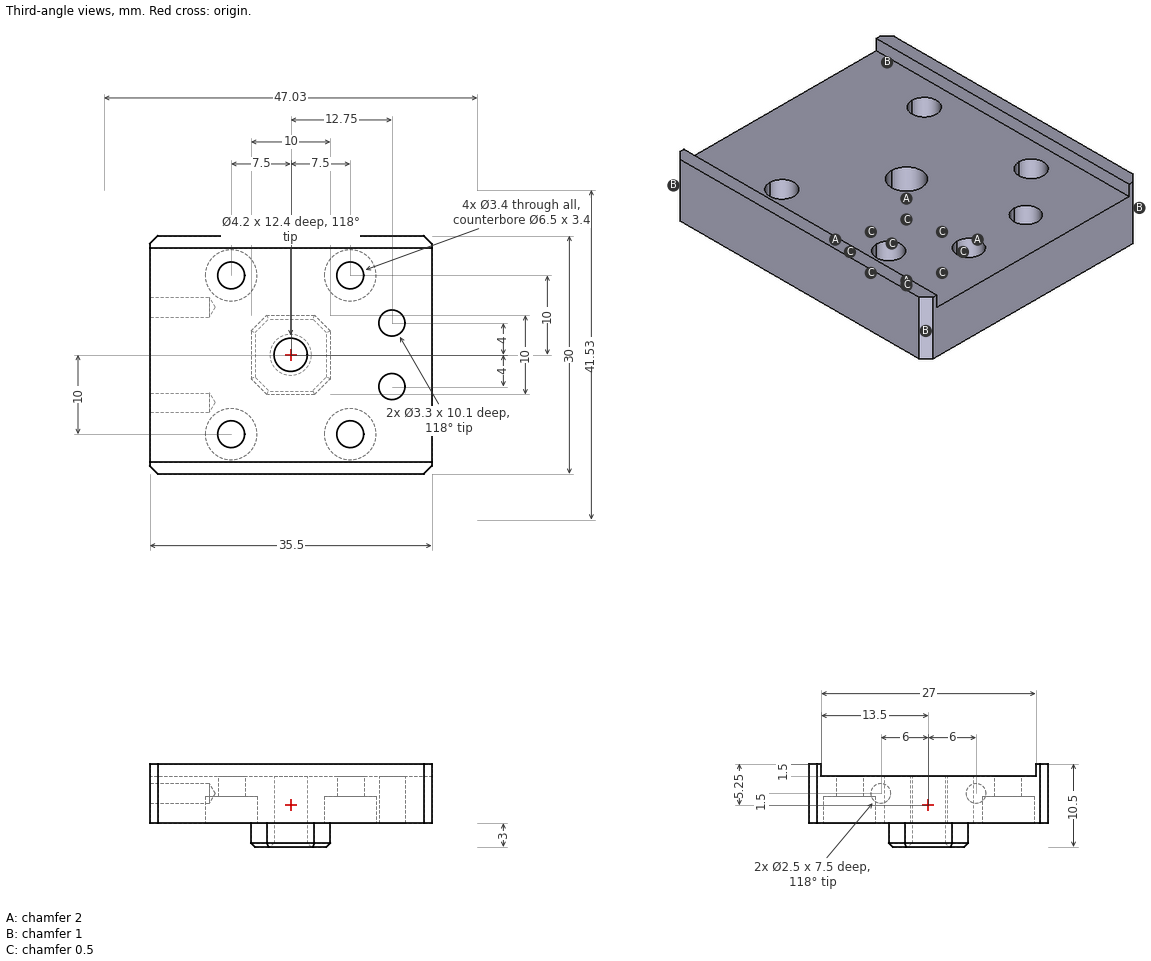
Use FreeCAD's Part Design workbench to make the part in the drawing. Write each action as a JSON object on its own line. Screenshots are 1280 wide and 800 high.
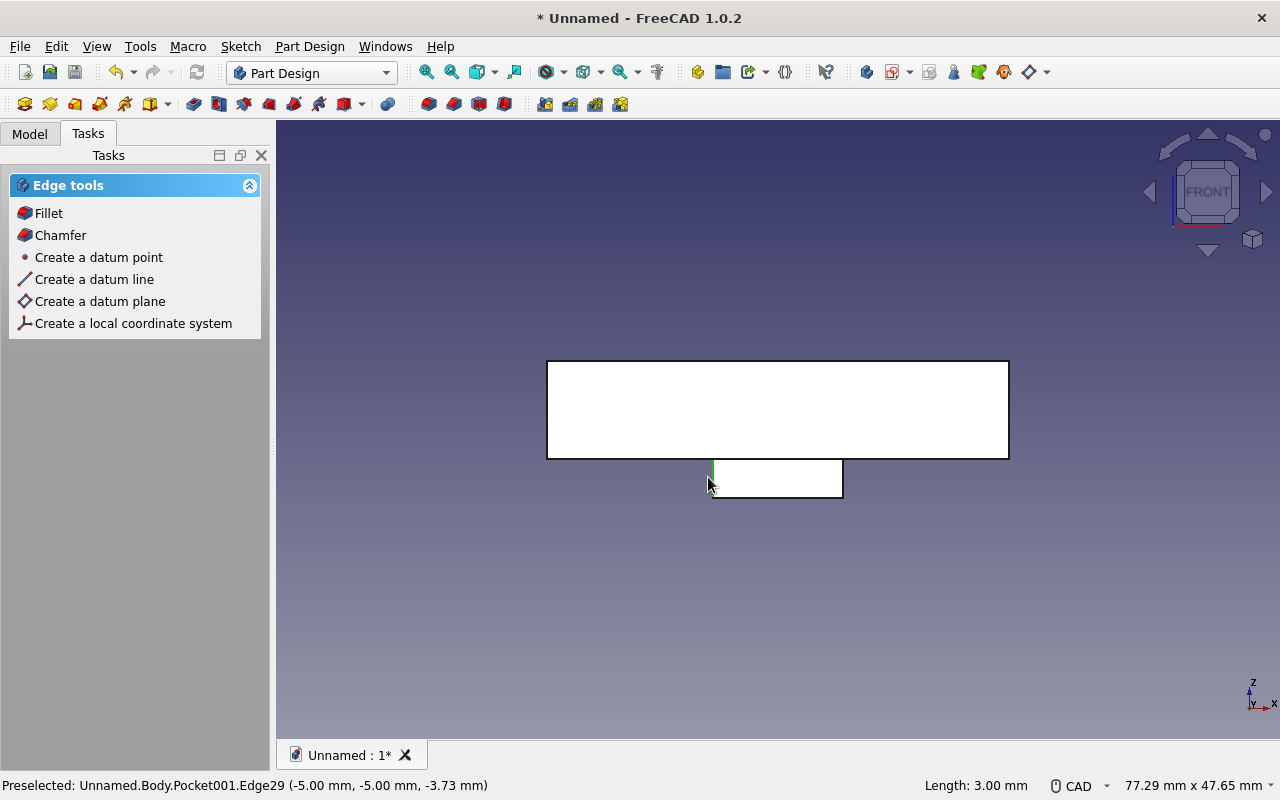
{"action": "left_click", "coordinate": [843, 477], "text": "ctrl"}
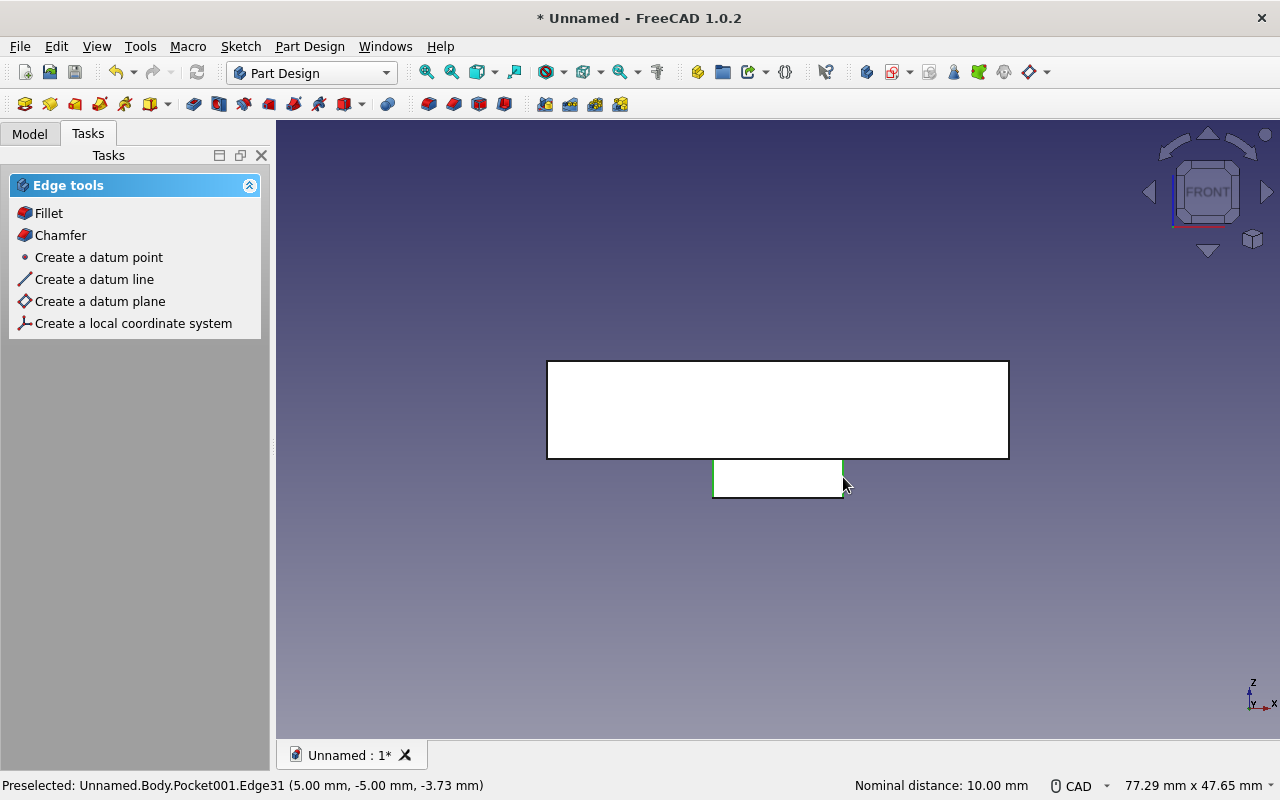
{"action": "key", "text": "3"}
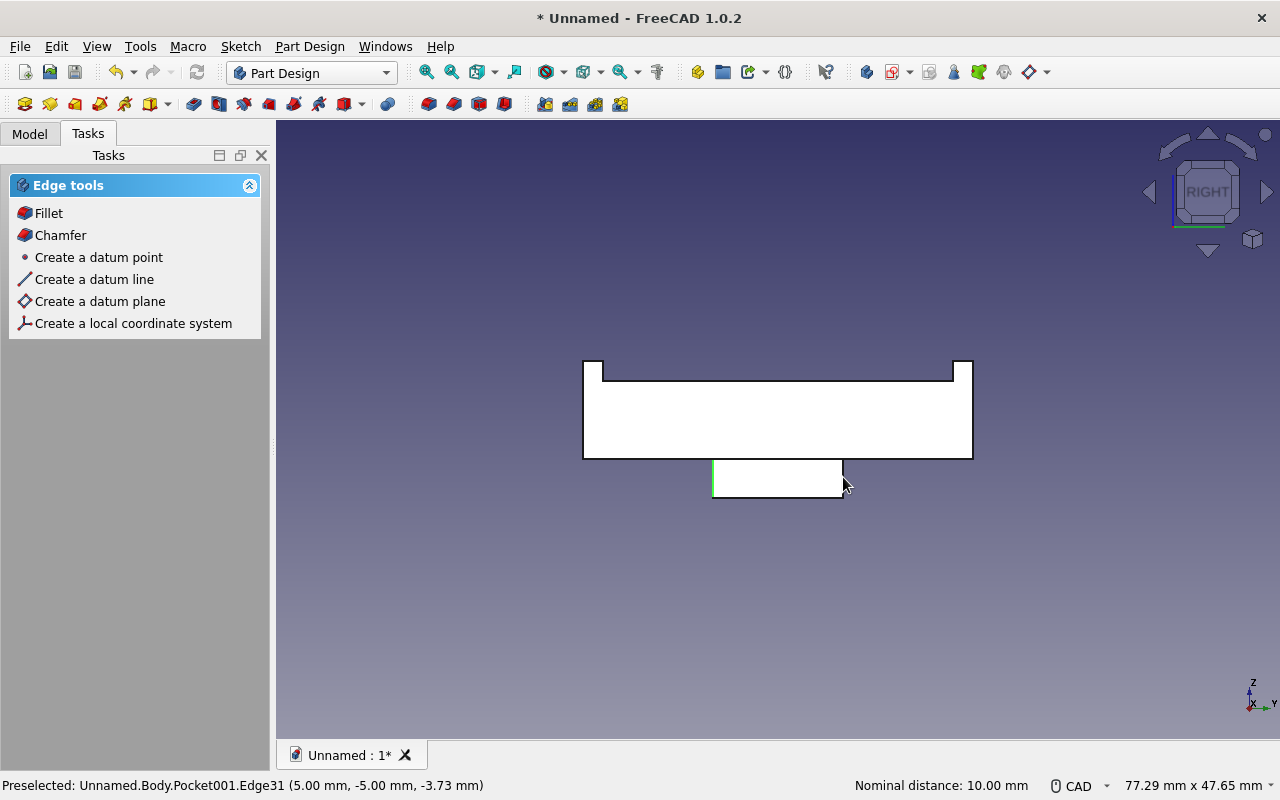
{"action": "key", "text": "v f"}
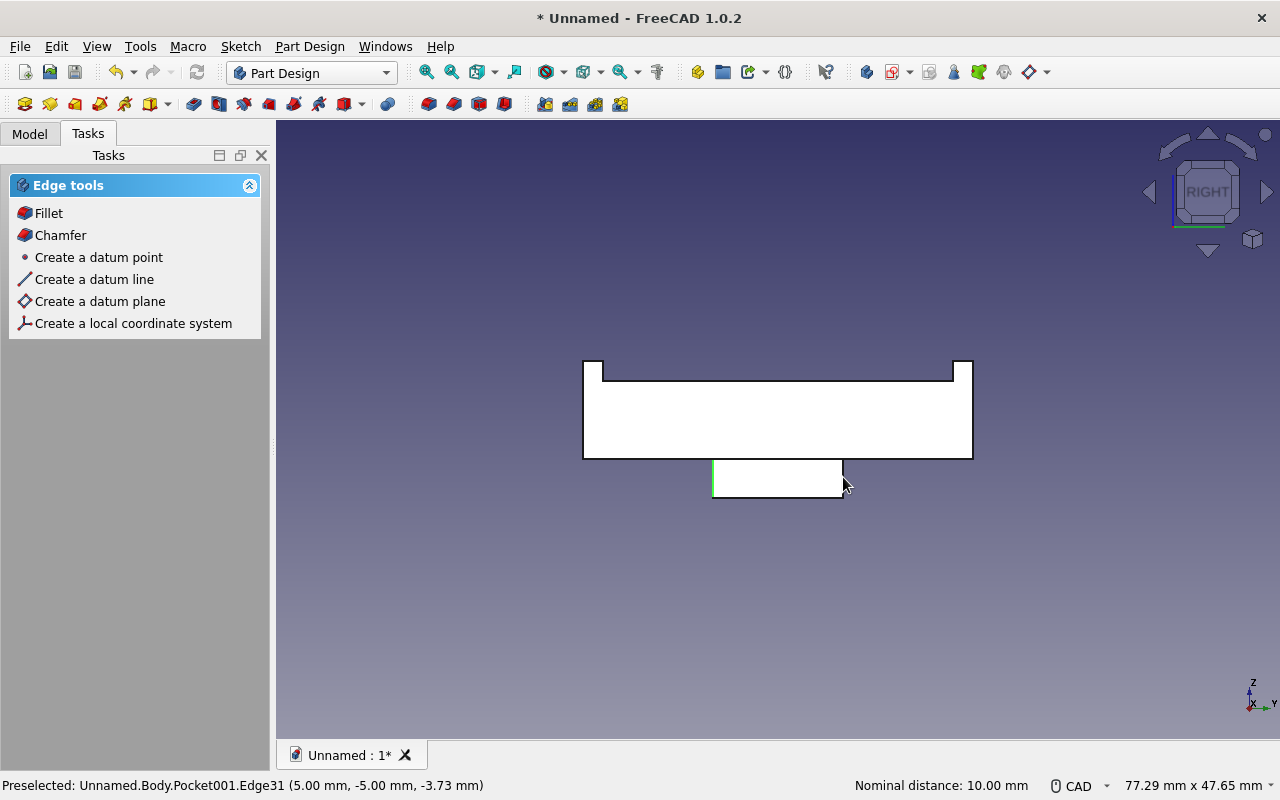
{"action": "left_click", "coordinate": [843, 477], "text": "ctrl"}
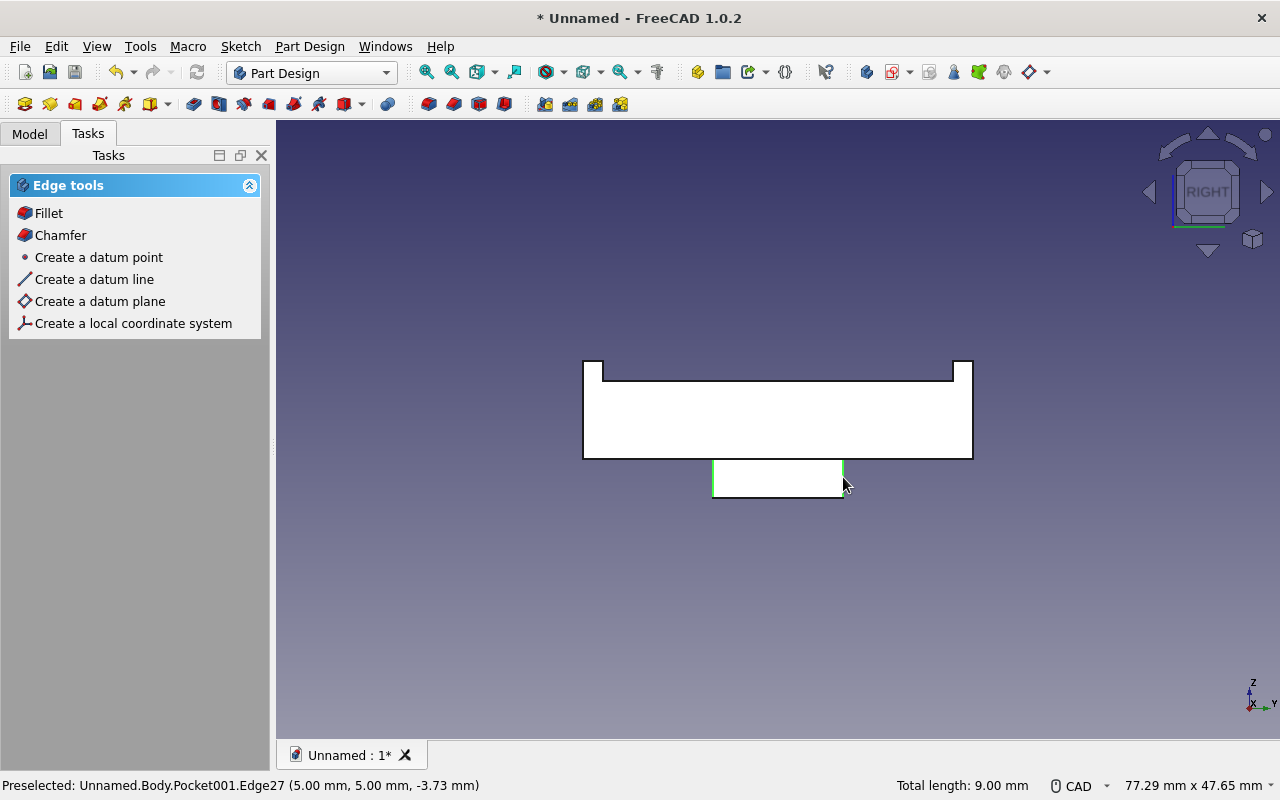
{"action": "key", "text": "5"}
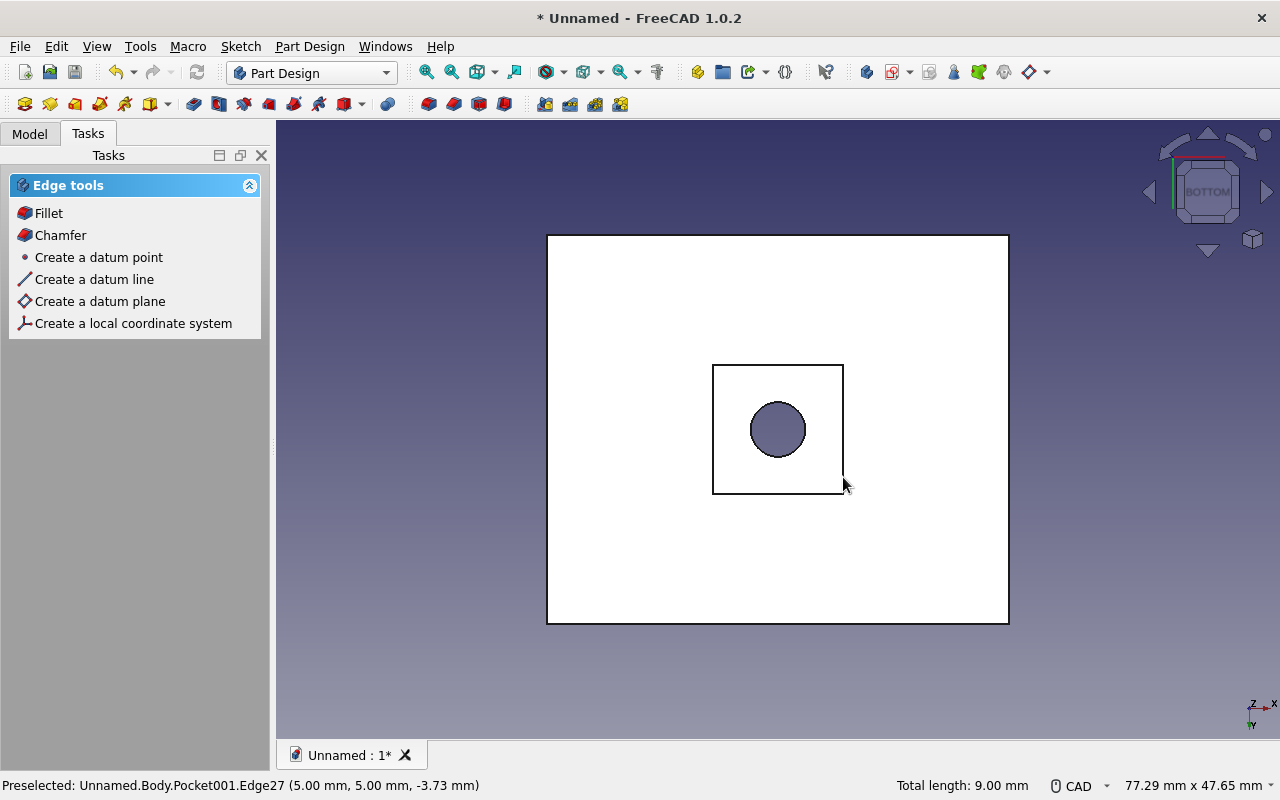
{"action": "key", "text": "4"}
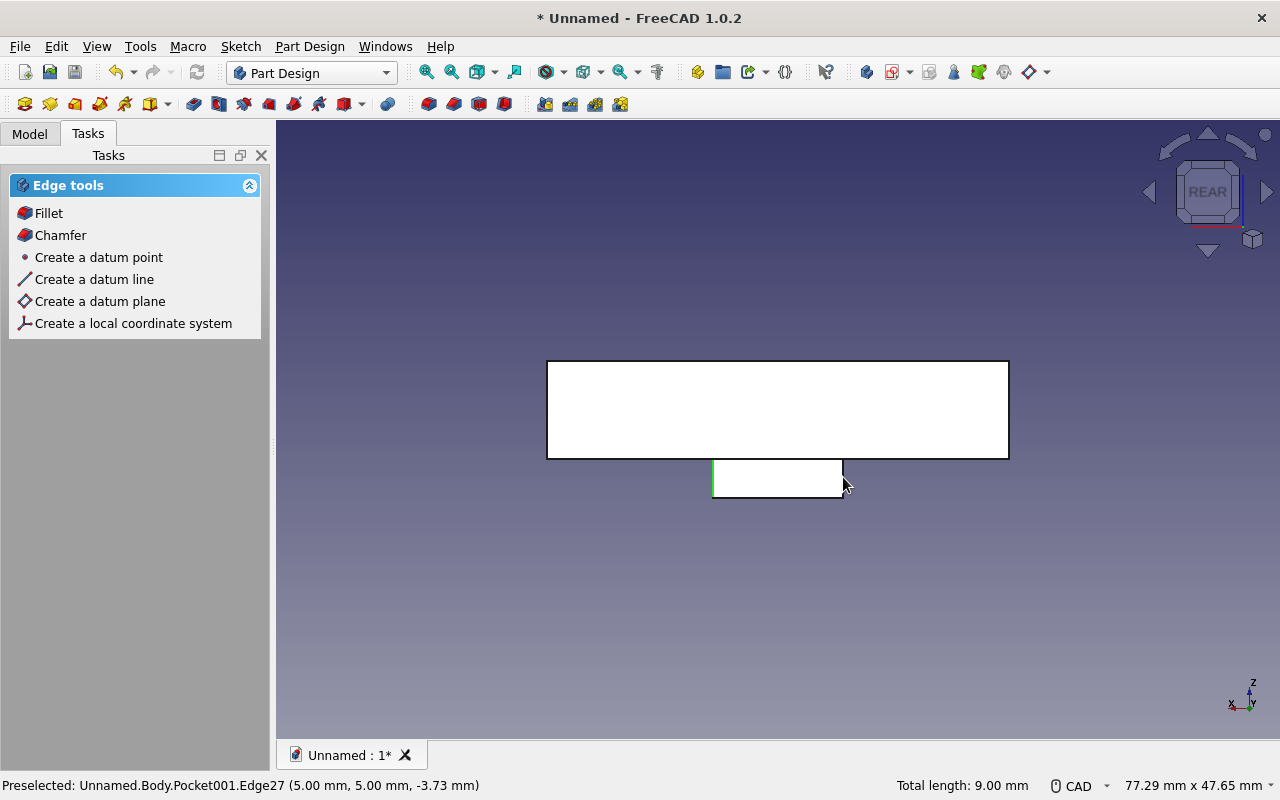
{"action": "left_click", "coordinate": [843, 477], "text": "ctrl"}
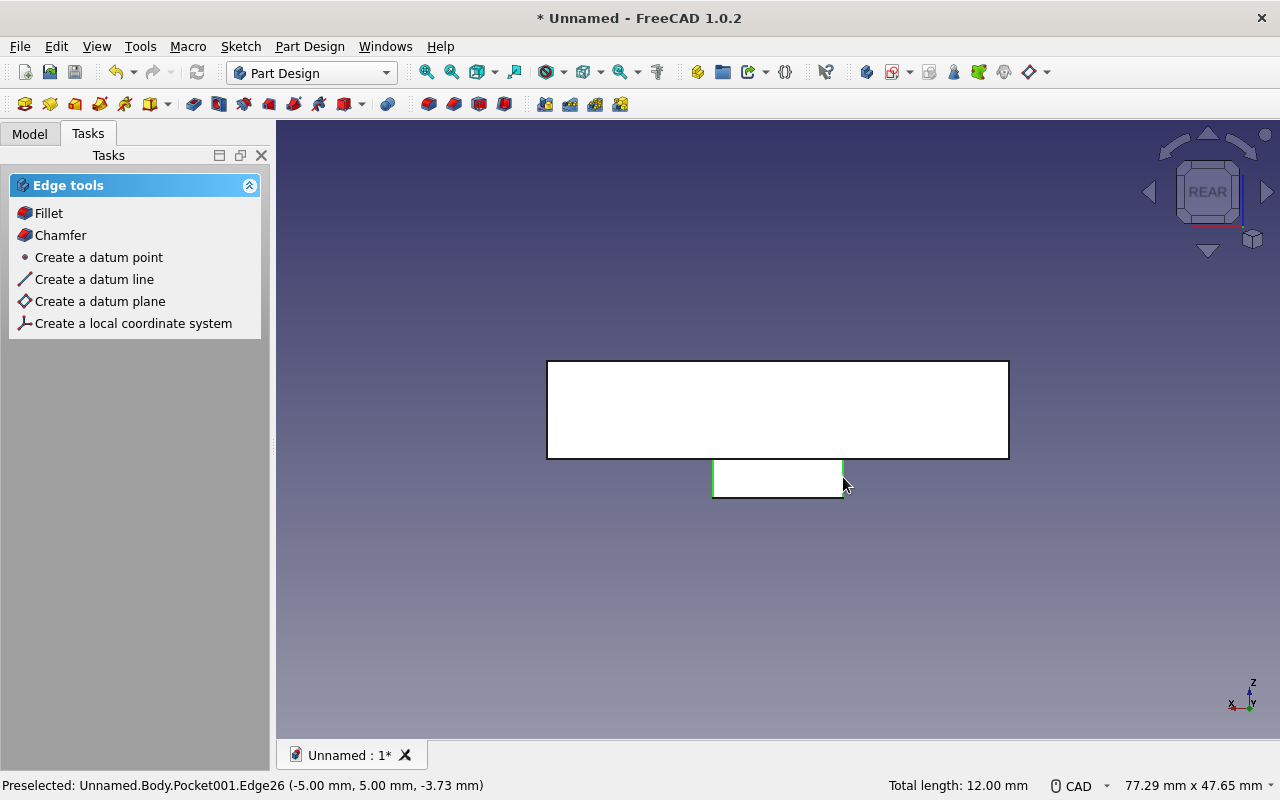
{"action": "left_click", "coordinate": [454, 104]}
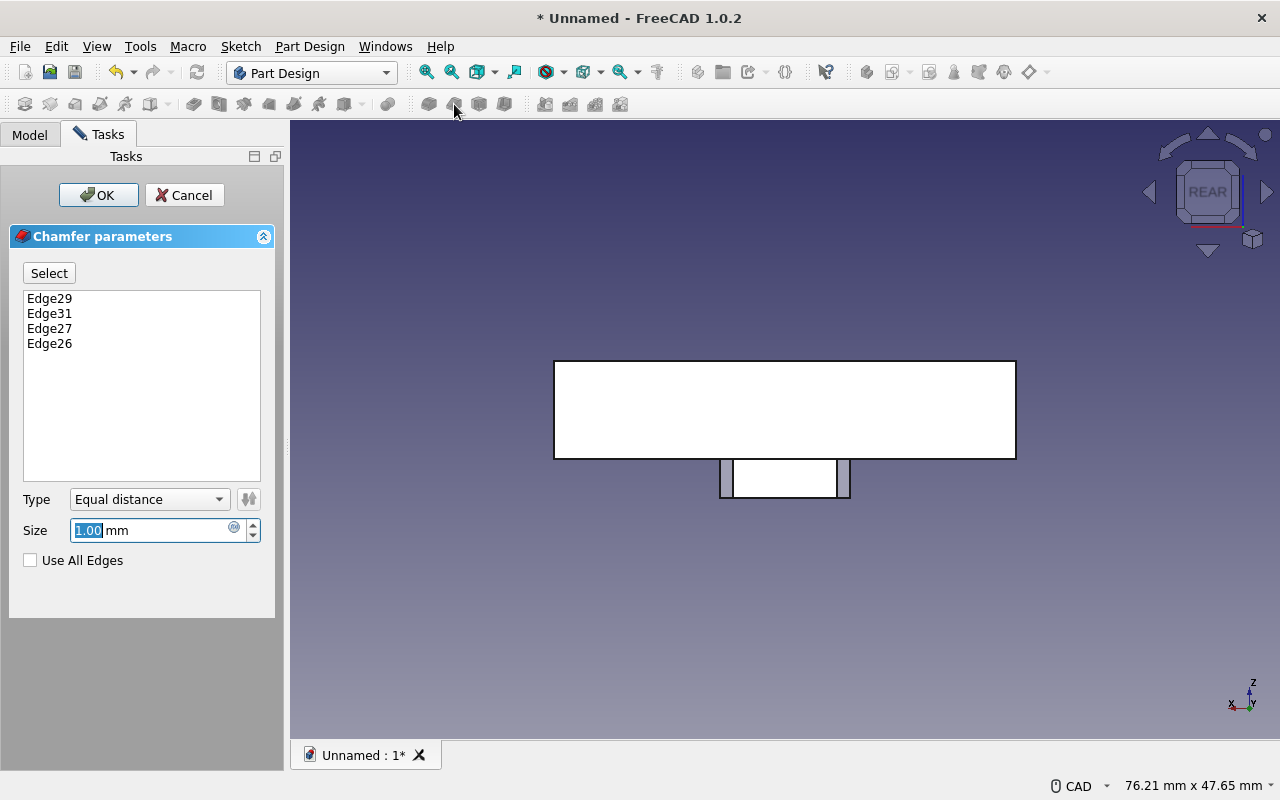
{"action": "type", "text": "2"}
{"action": "key", "text": "Tab"}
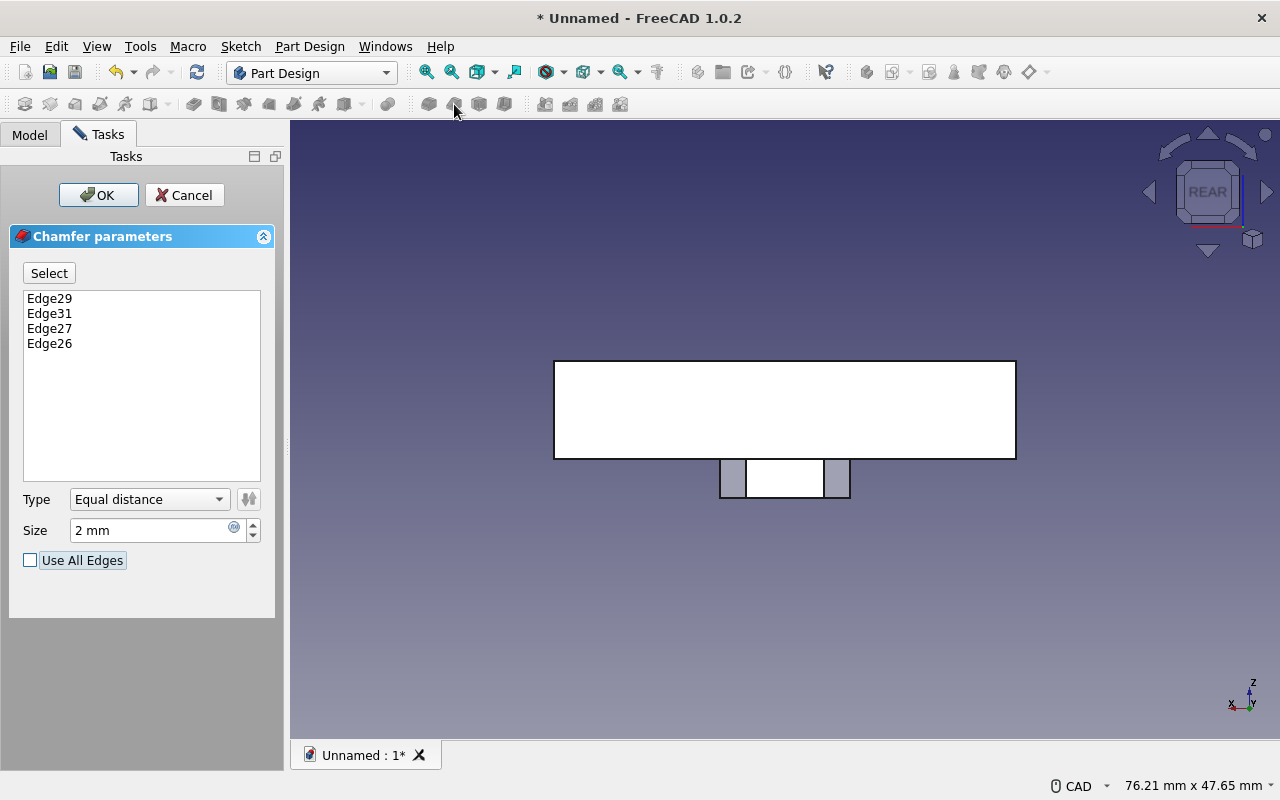
{"action": "left_click", "coordinate": [99, 195]}